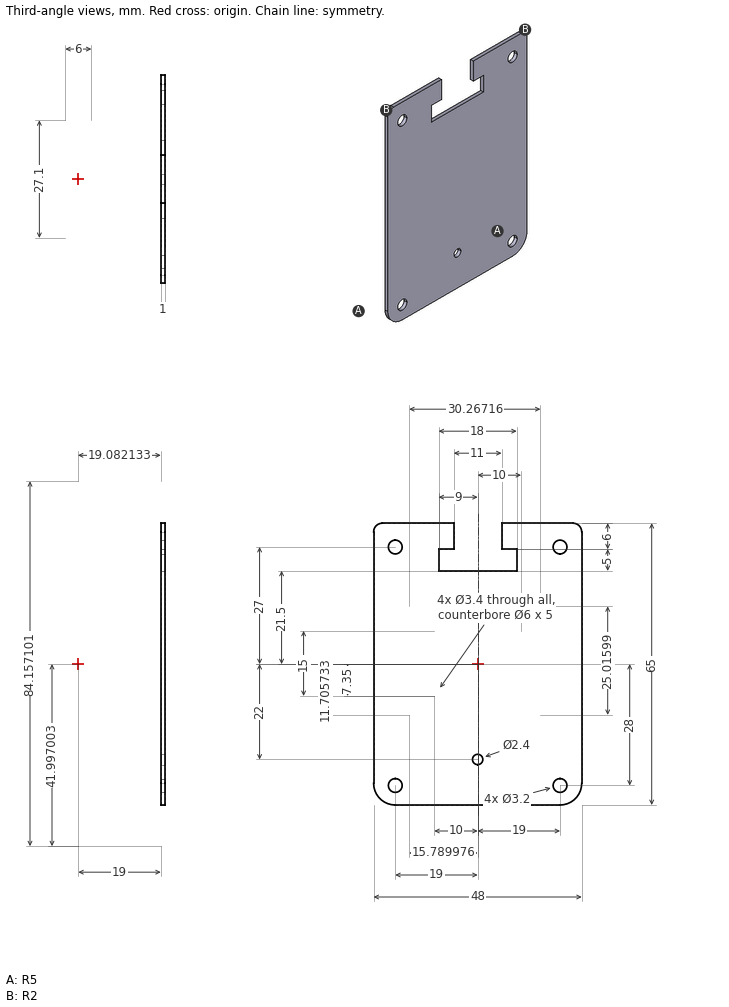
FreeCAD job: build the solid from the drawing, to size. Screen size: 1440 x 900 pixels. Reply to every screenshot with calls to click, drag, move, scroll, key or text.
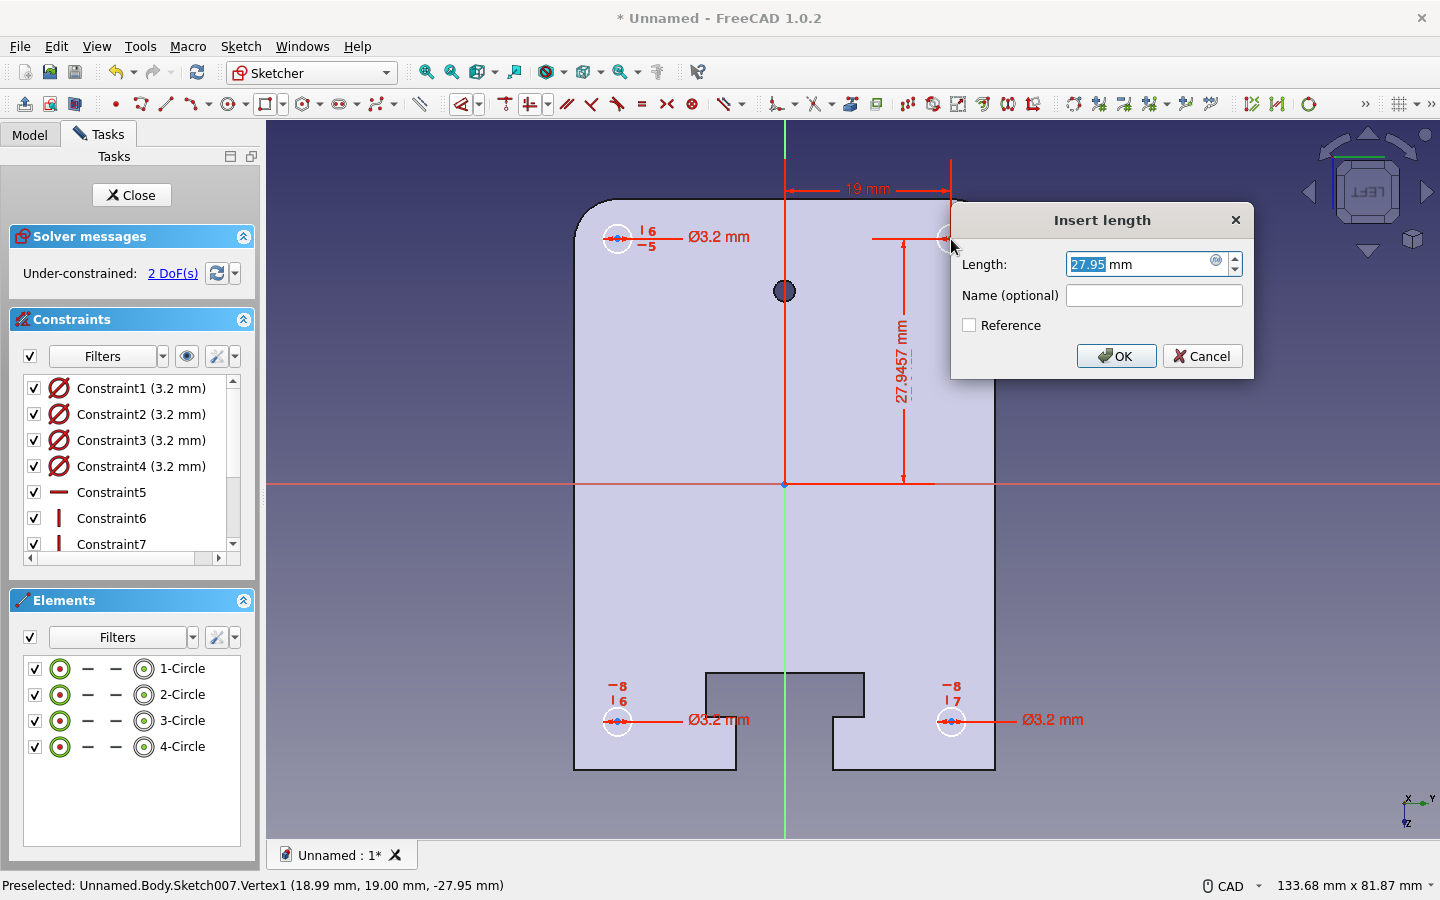
text(28)
key(Return)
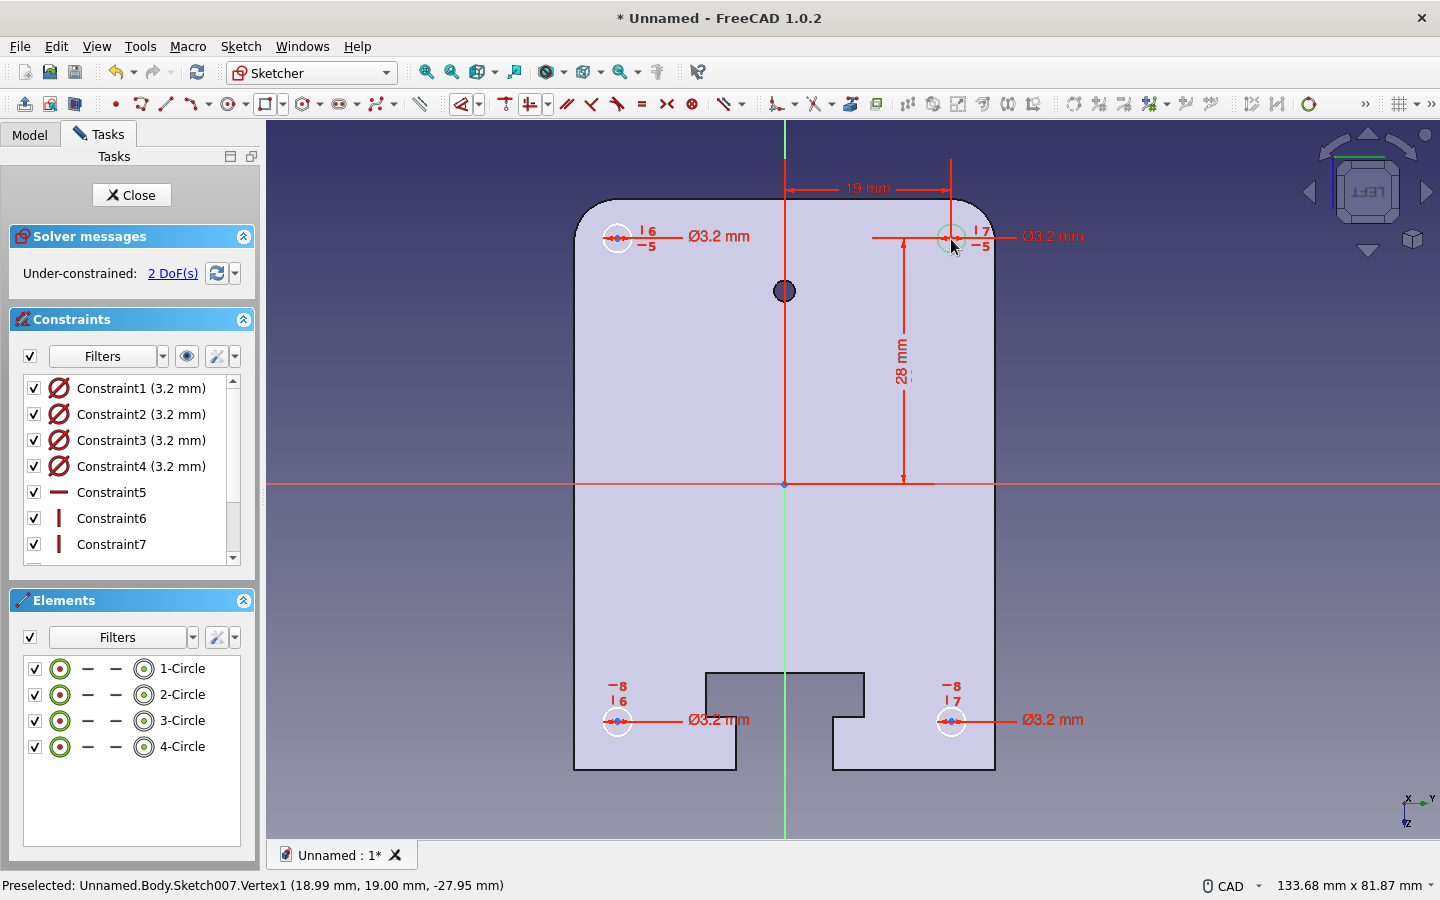
click(618, 238)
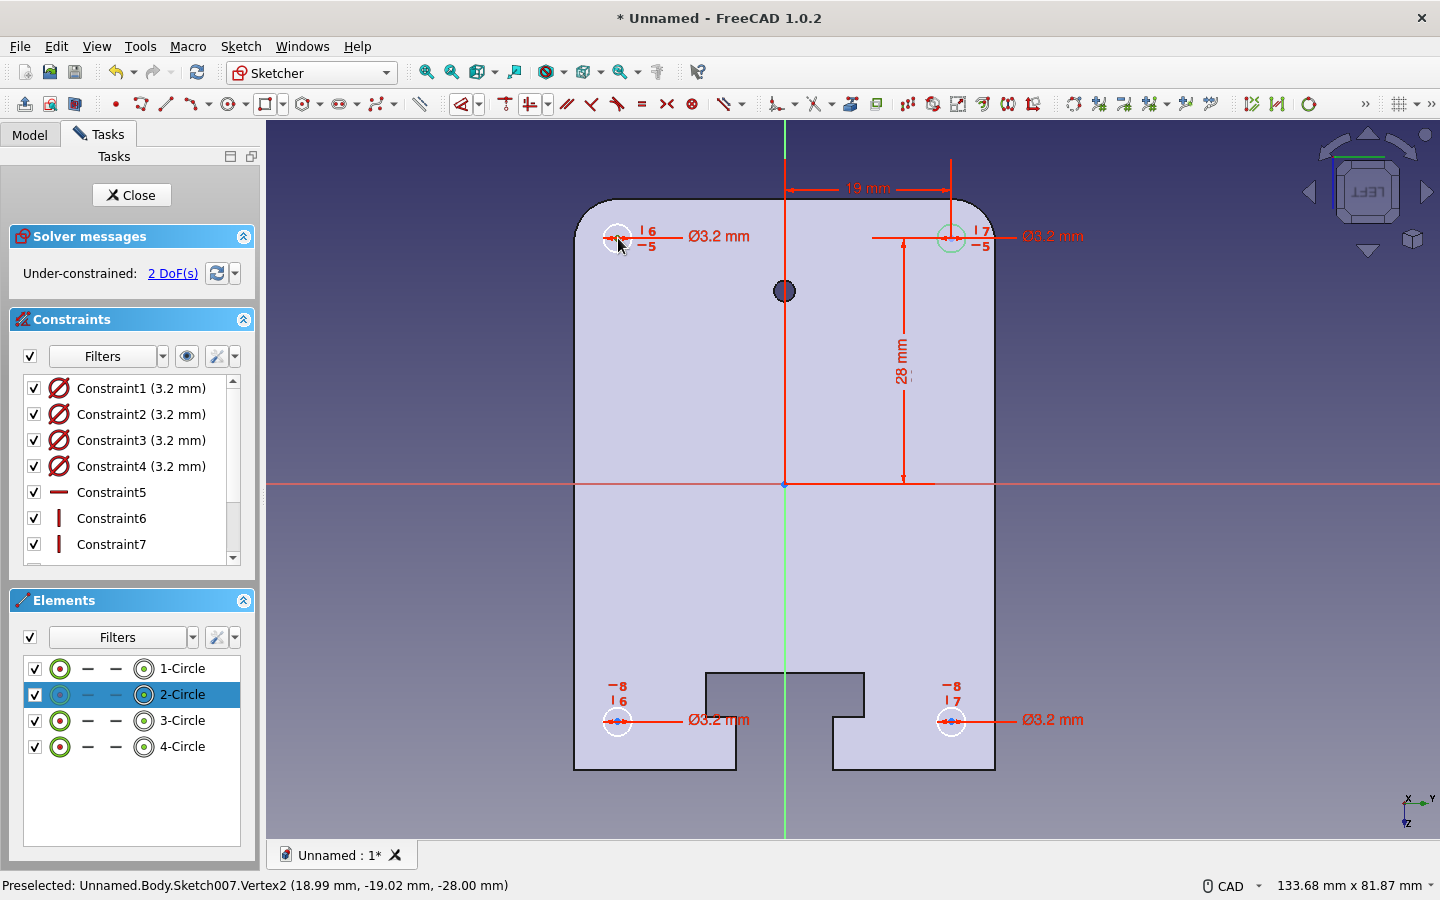
click(478, 104)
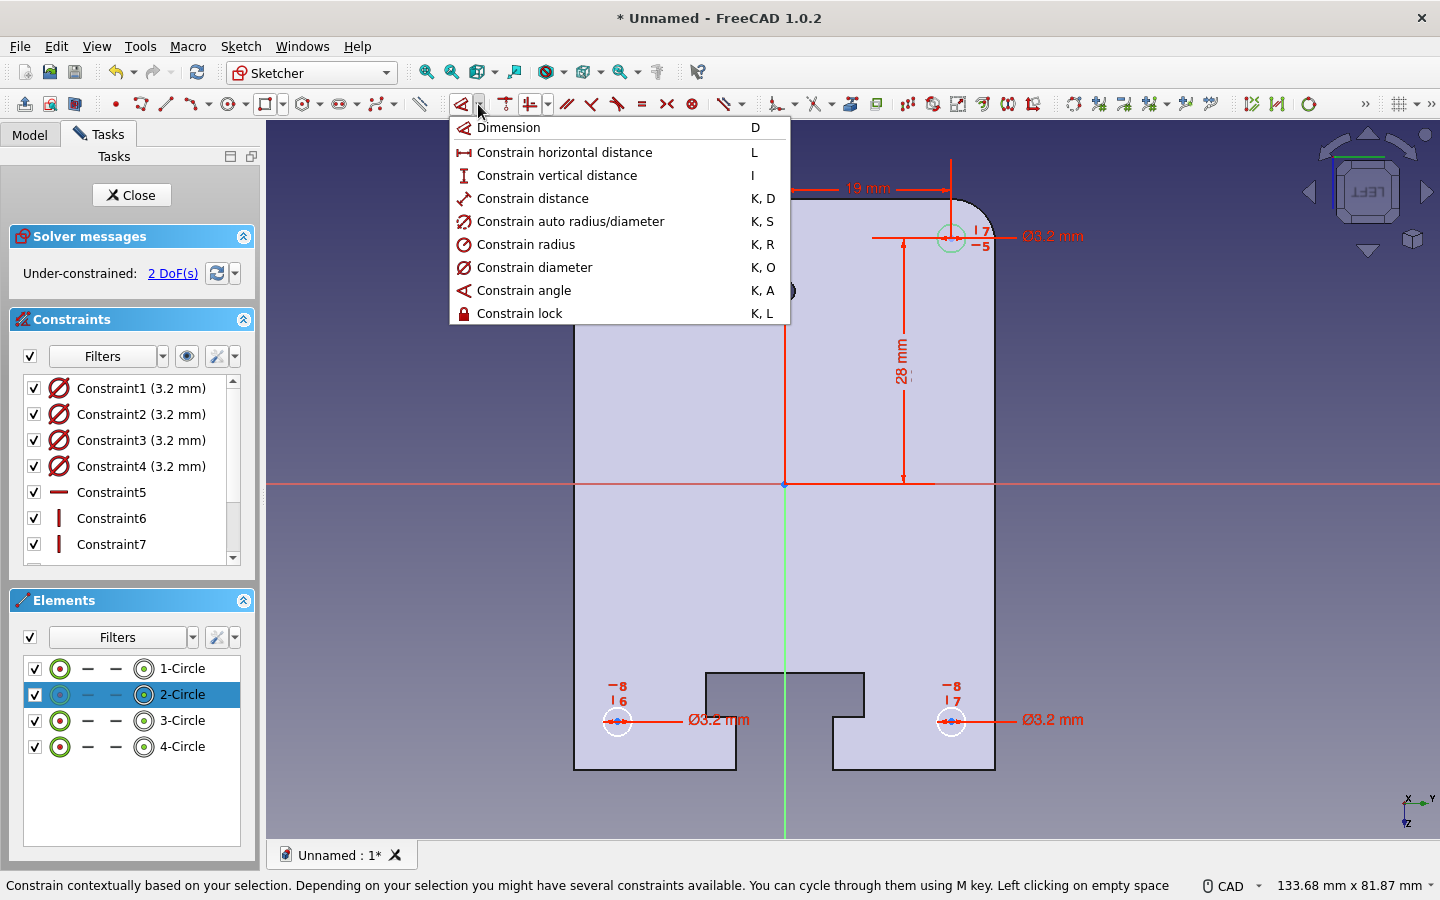
click(620, 152)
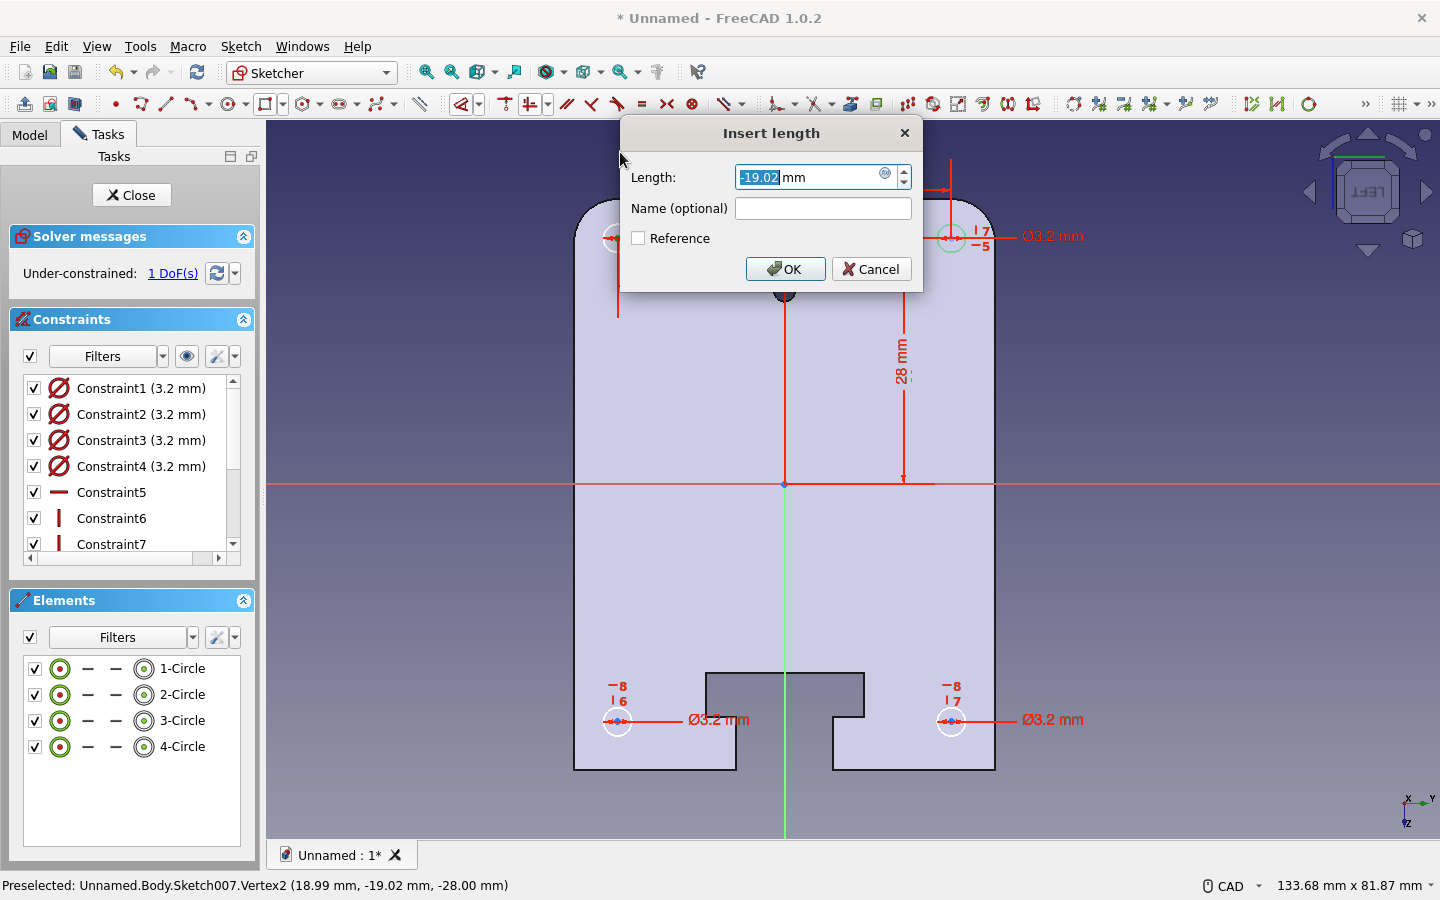
text(-19)
key(Return)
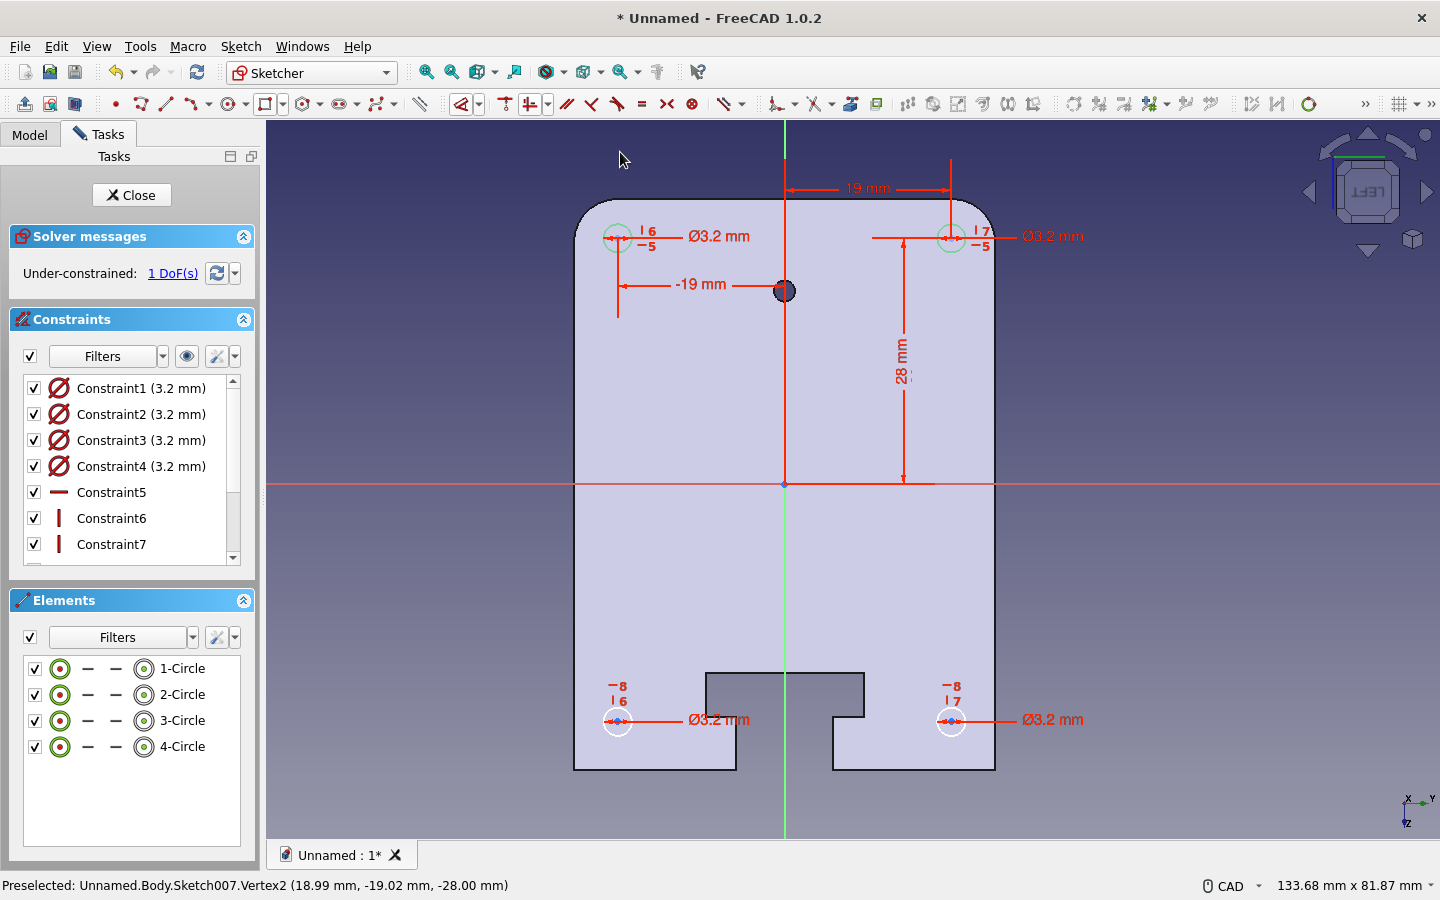
click(618, 722)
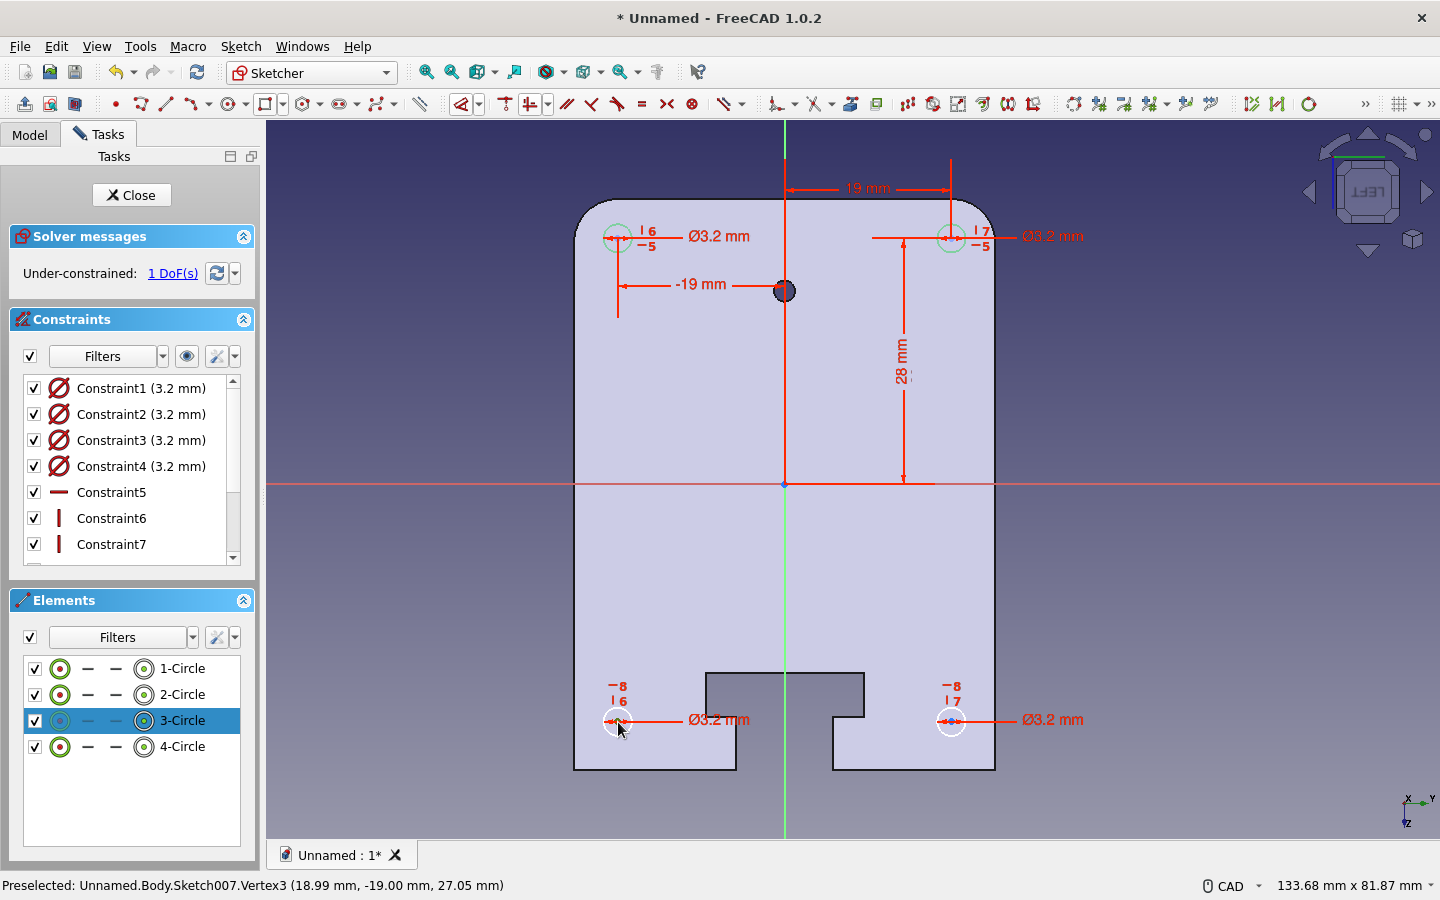
key(i)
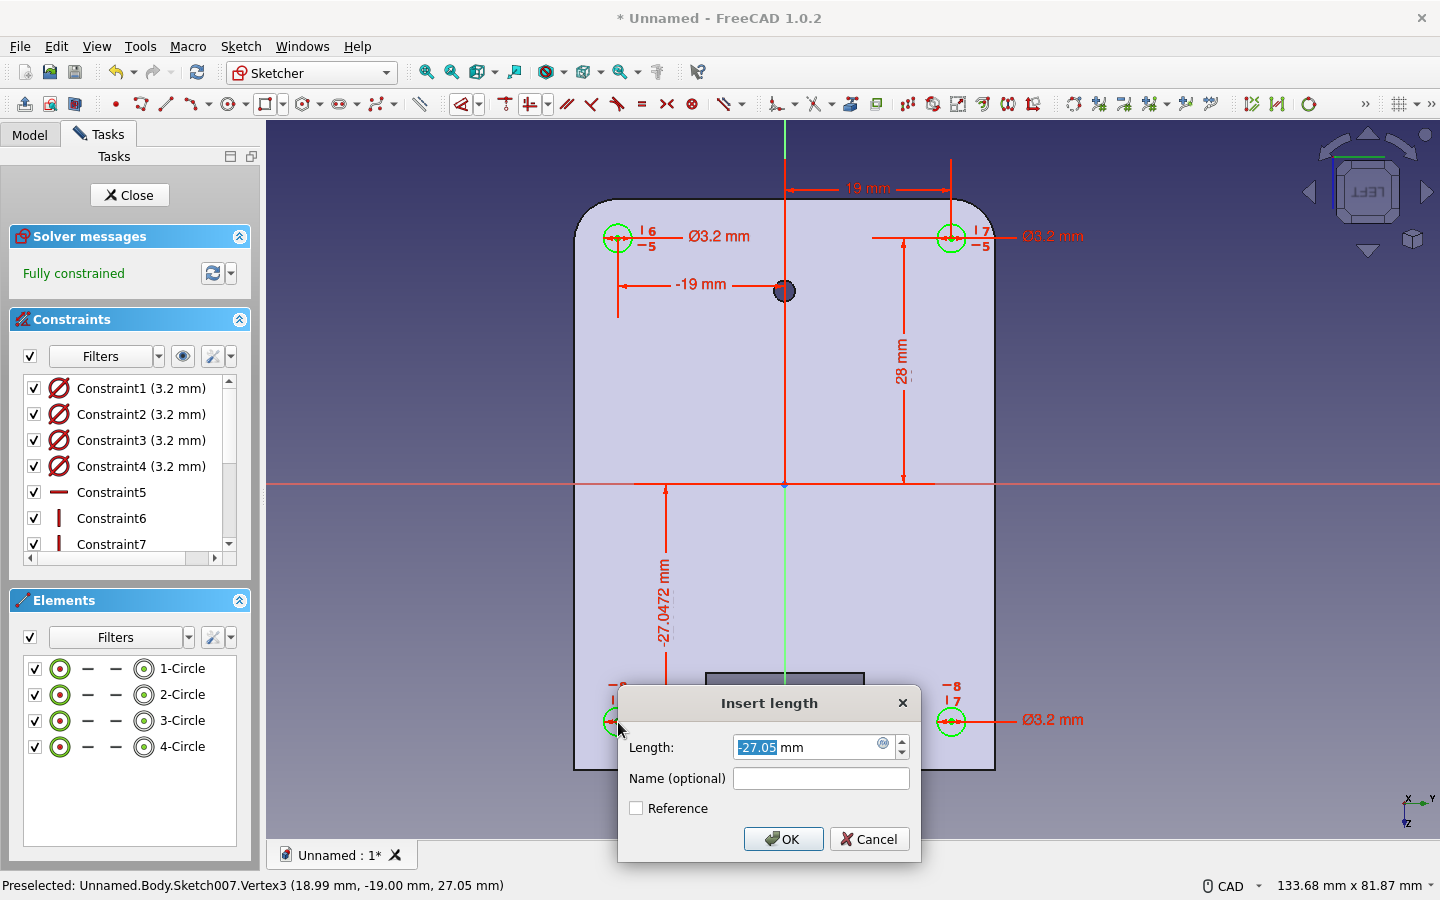
text(-27)
key(Return)